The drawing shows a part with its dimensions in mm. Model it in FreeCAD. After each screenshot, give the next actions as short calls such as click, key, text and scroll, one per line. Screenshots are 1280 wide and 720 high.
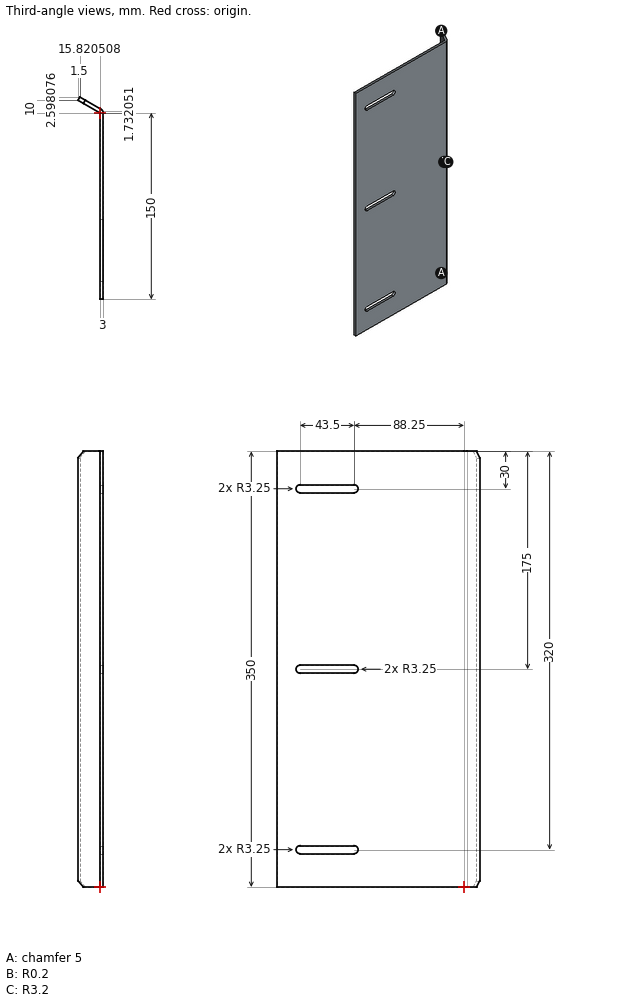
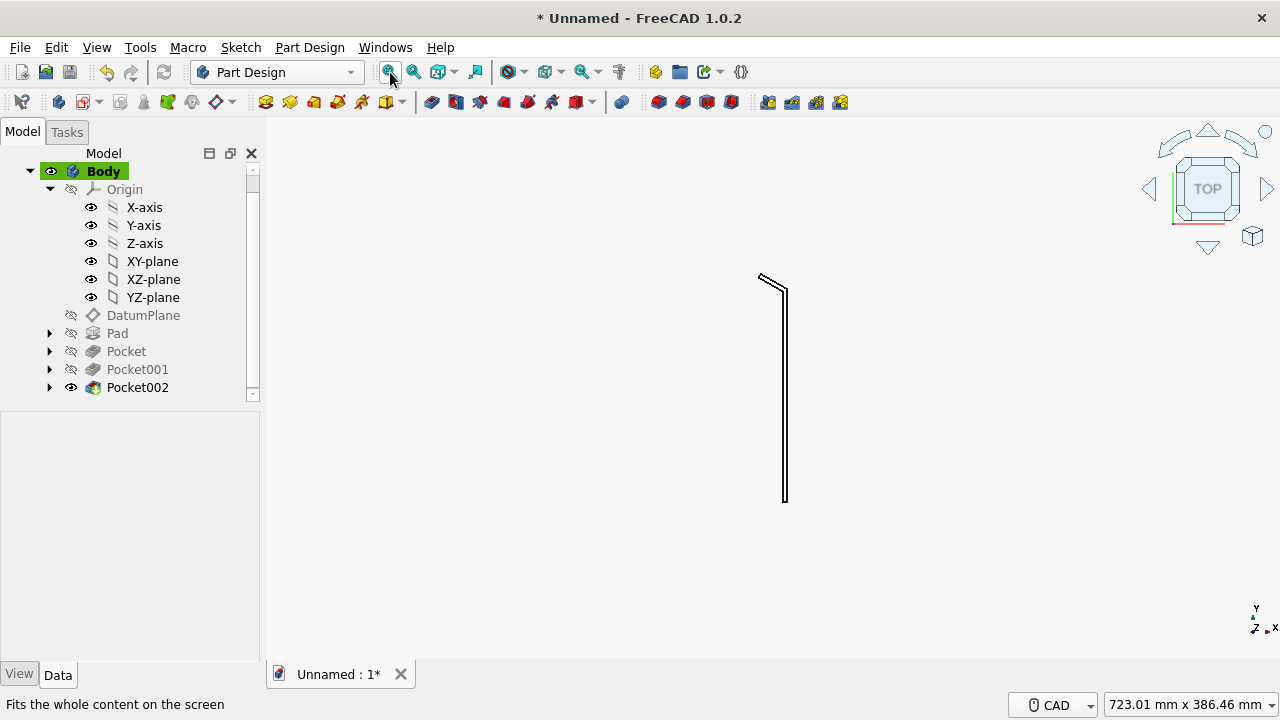
scroll(760, 275, up, 12)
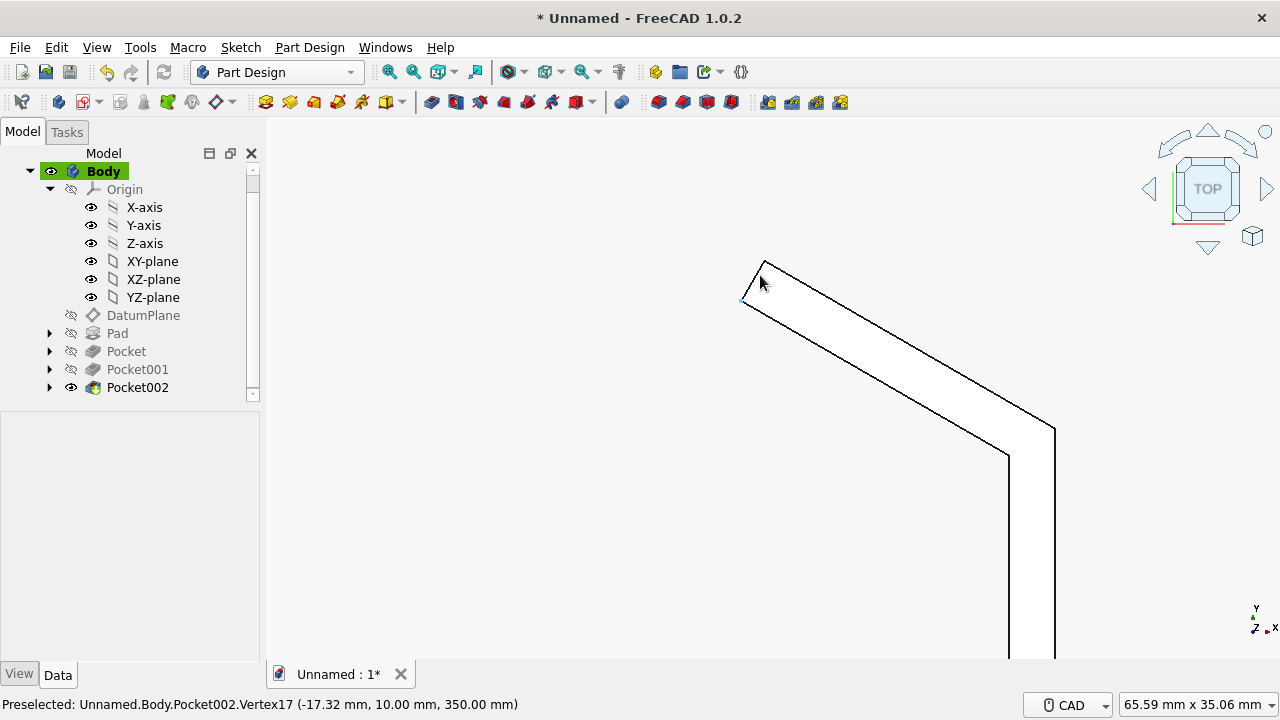
click(753, 280)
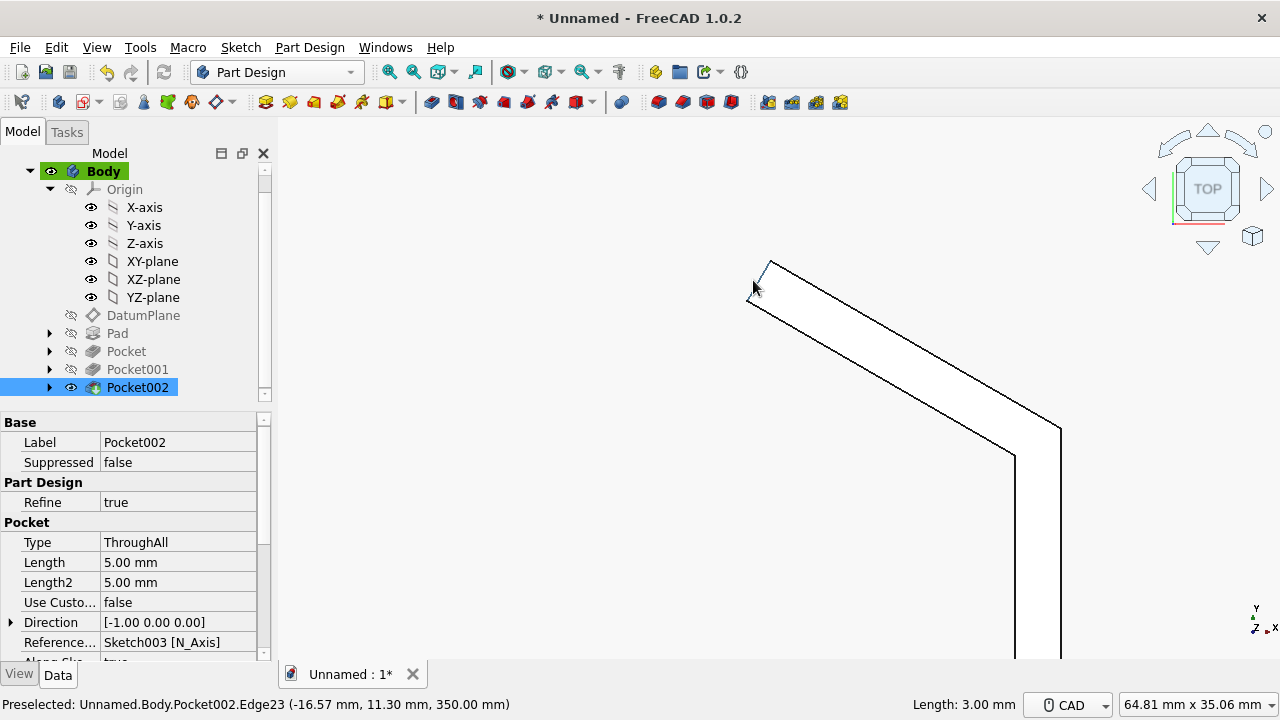
click(390, 72)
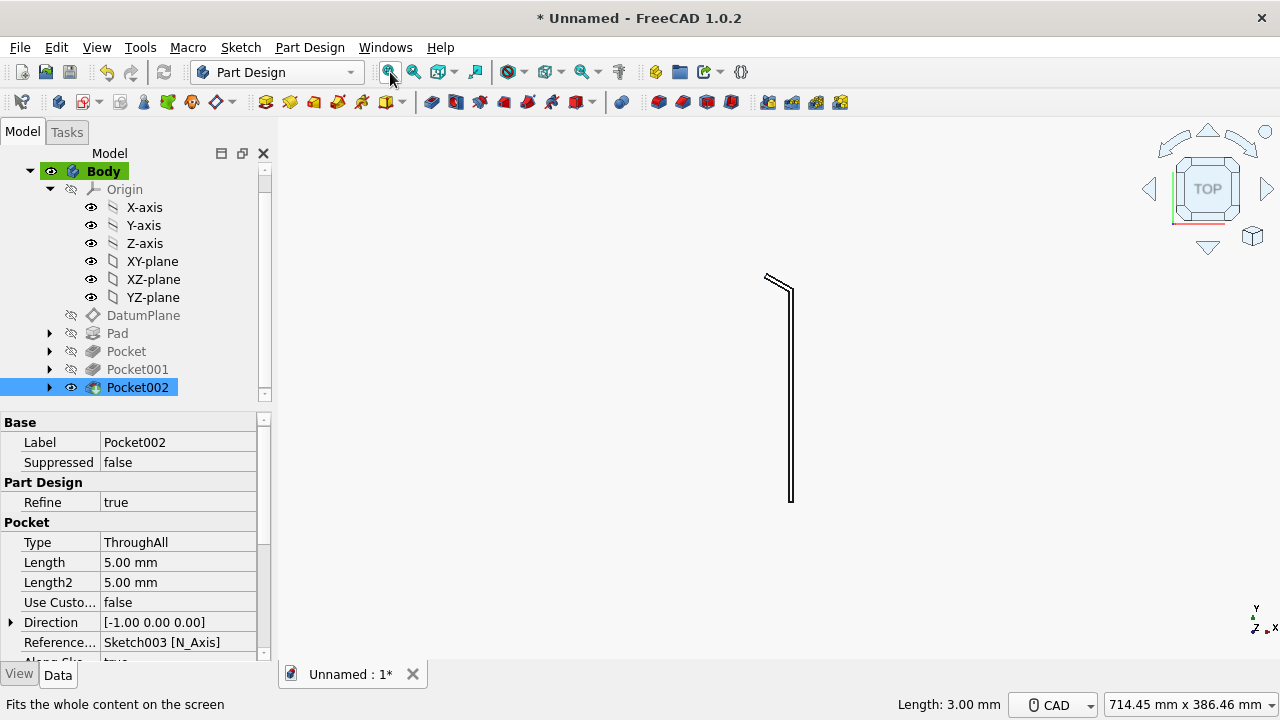
key(0)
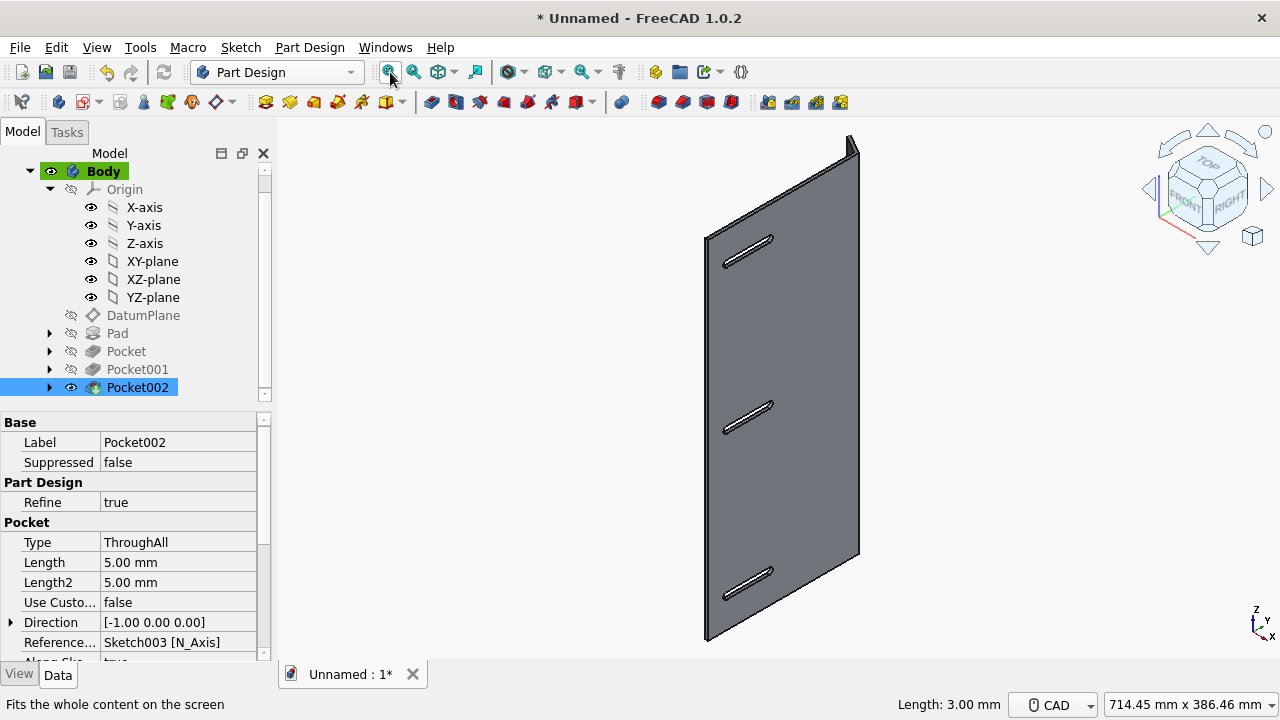
scroll(849, 536, up, 12)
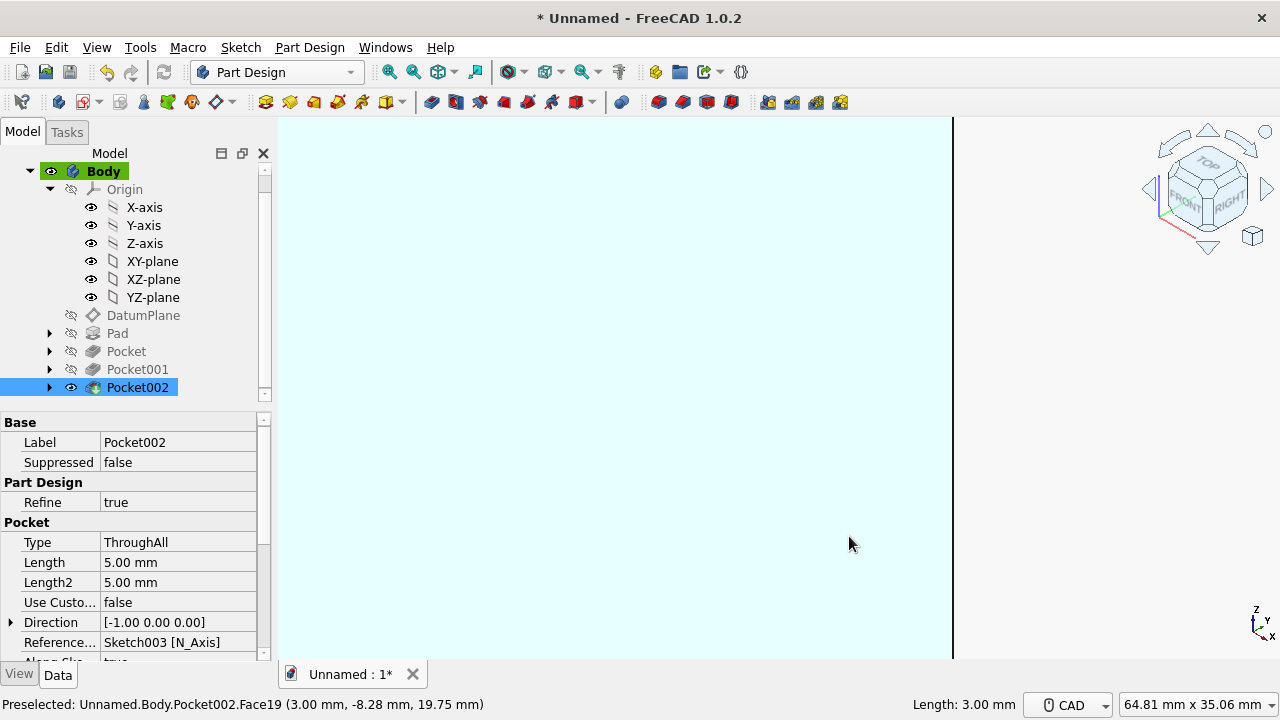
click(390, 72)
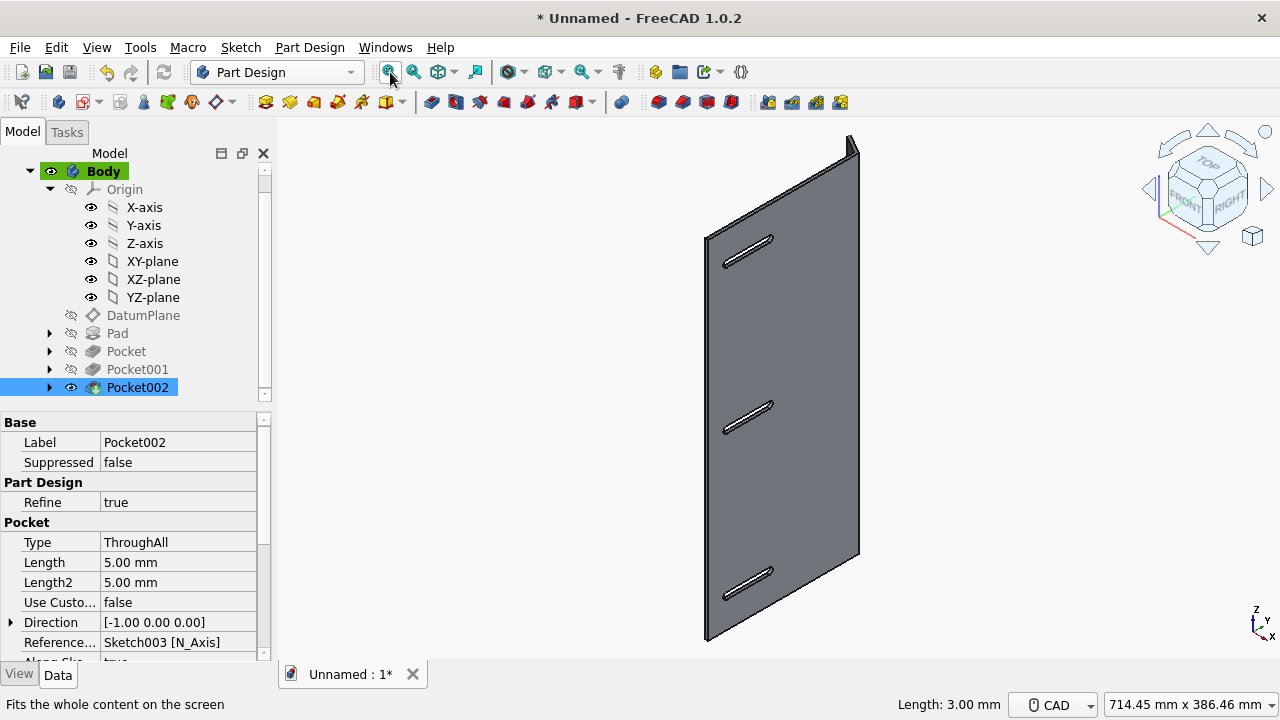
key(1)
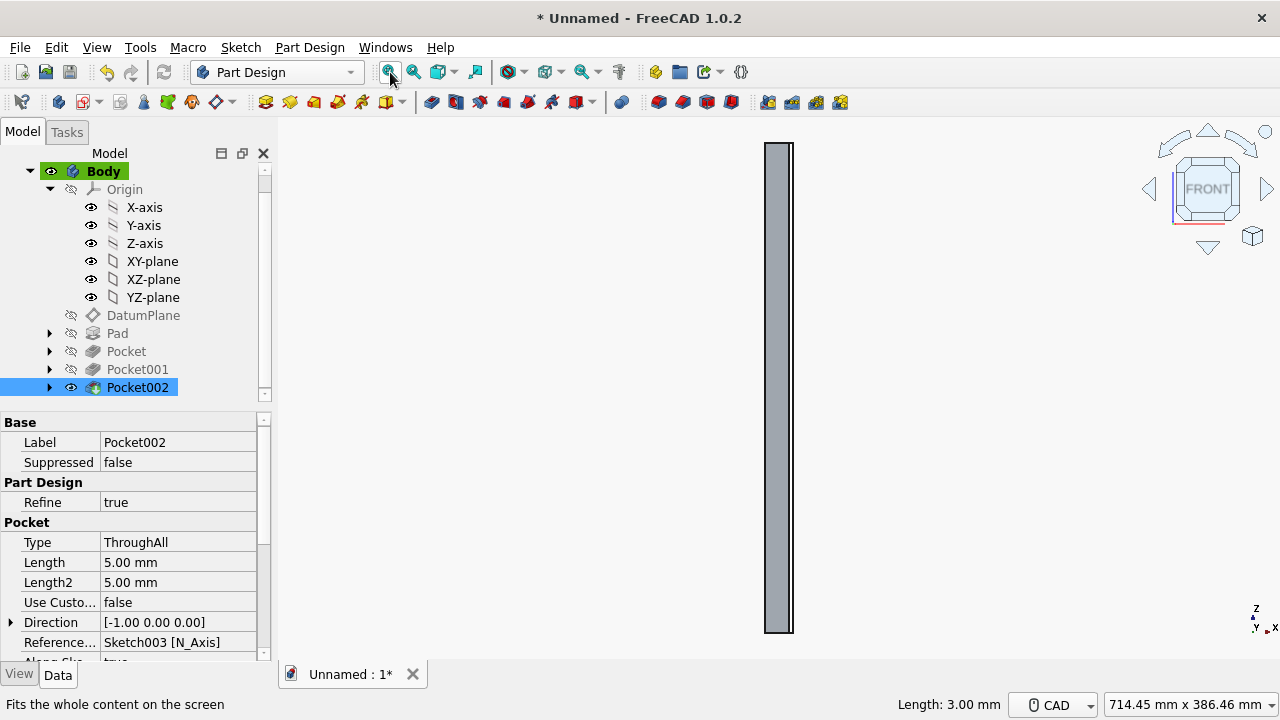
key(3)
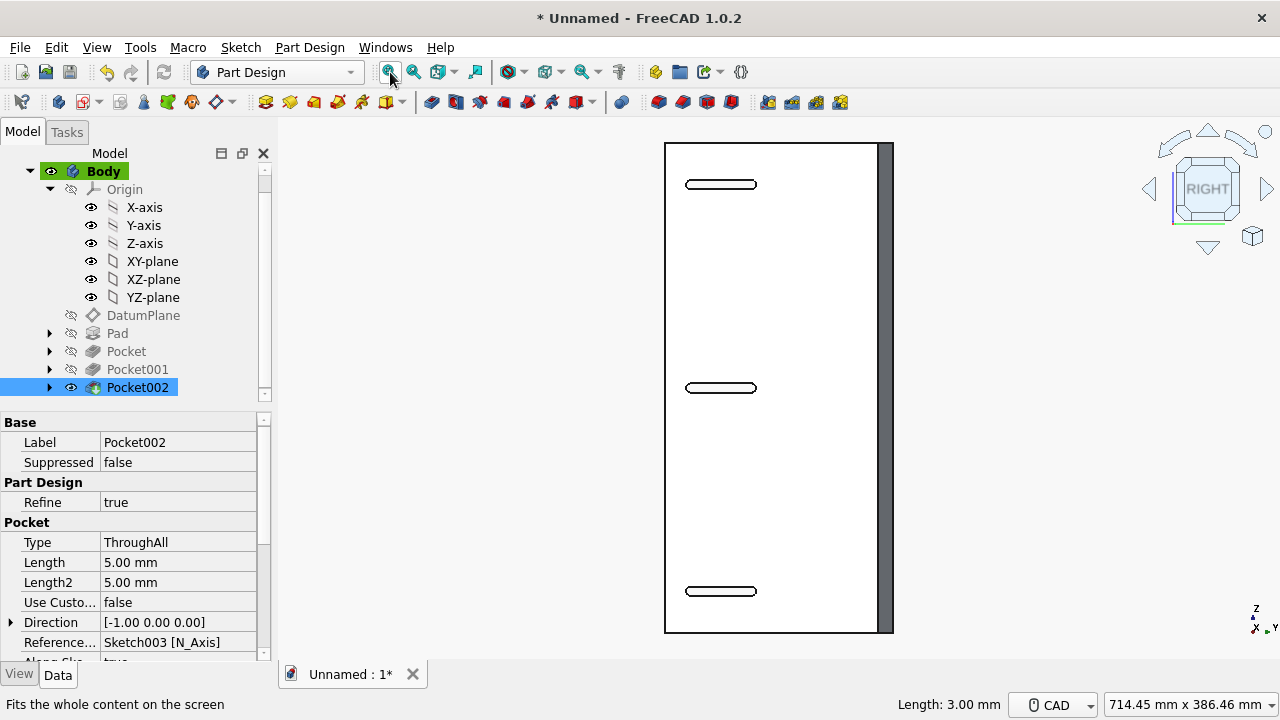
key(5)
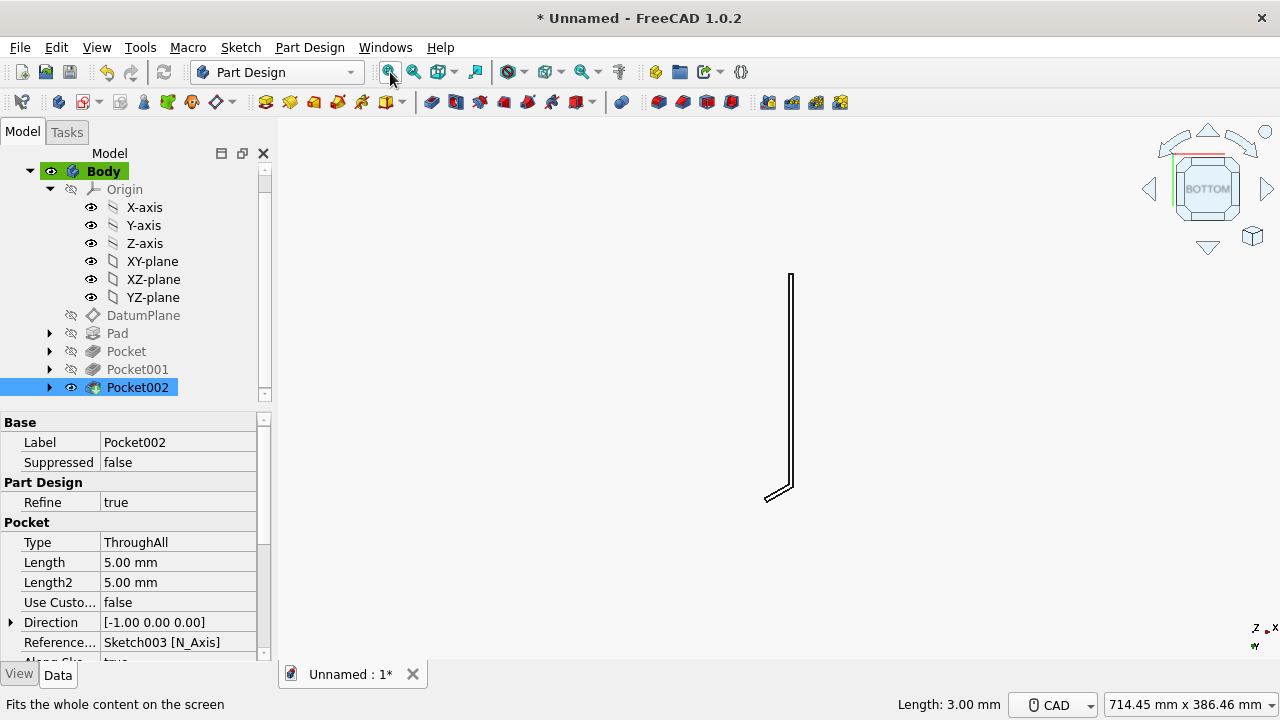
click(390, 72)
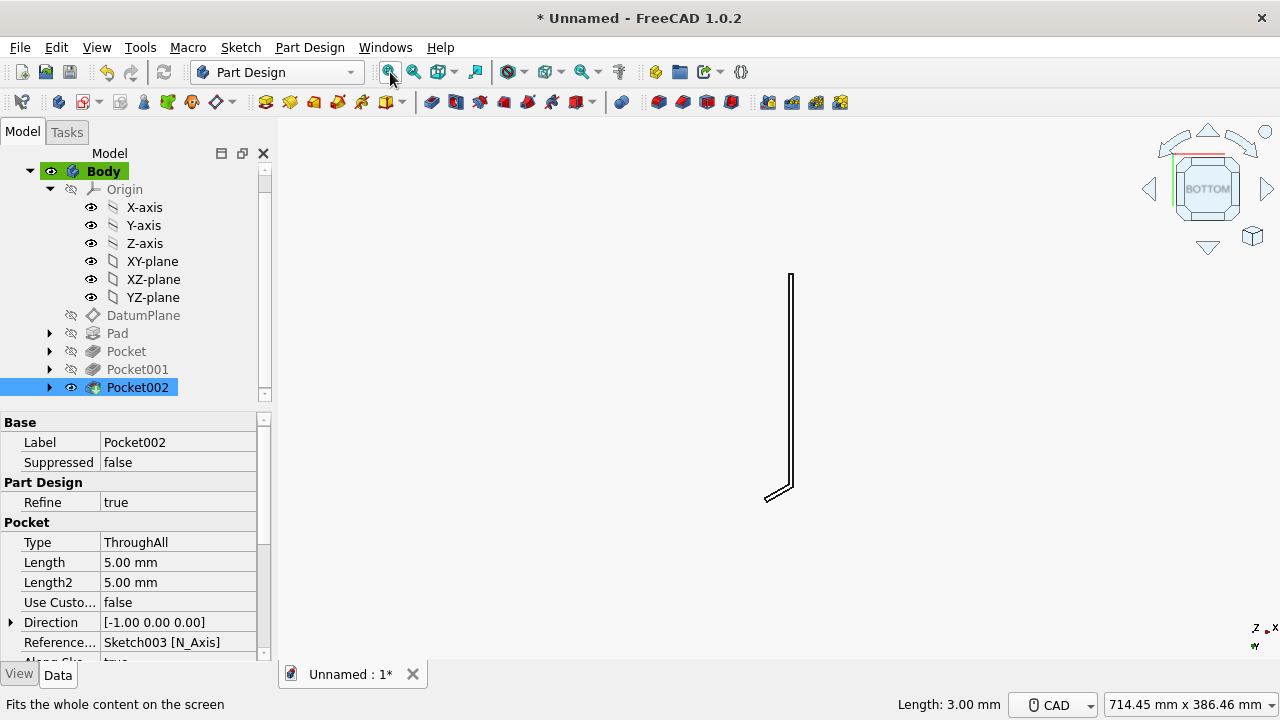
scroll(766, 499, up, 12)